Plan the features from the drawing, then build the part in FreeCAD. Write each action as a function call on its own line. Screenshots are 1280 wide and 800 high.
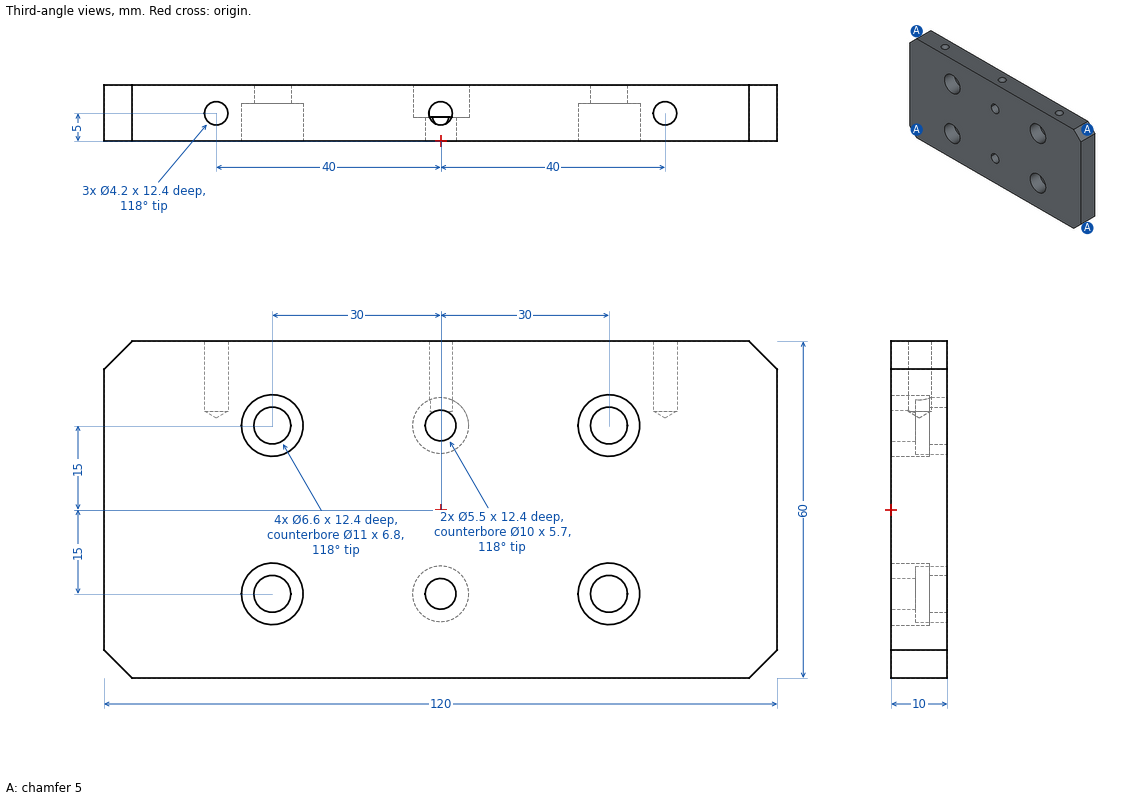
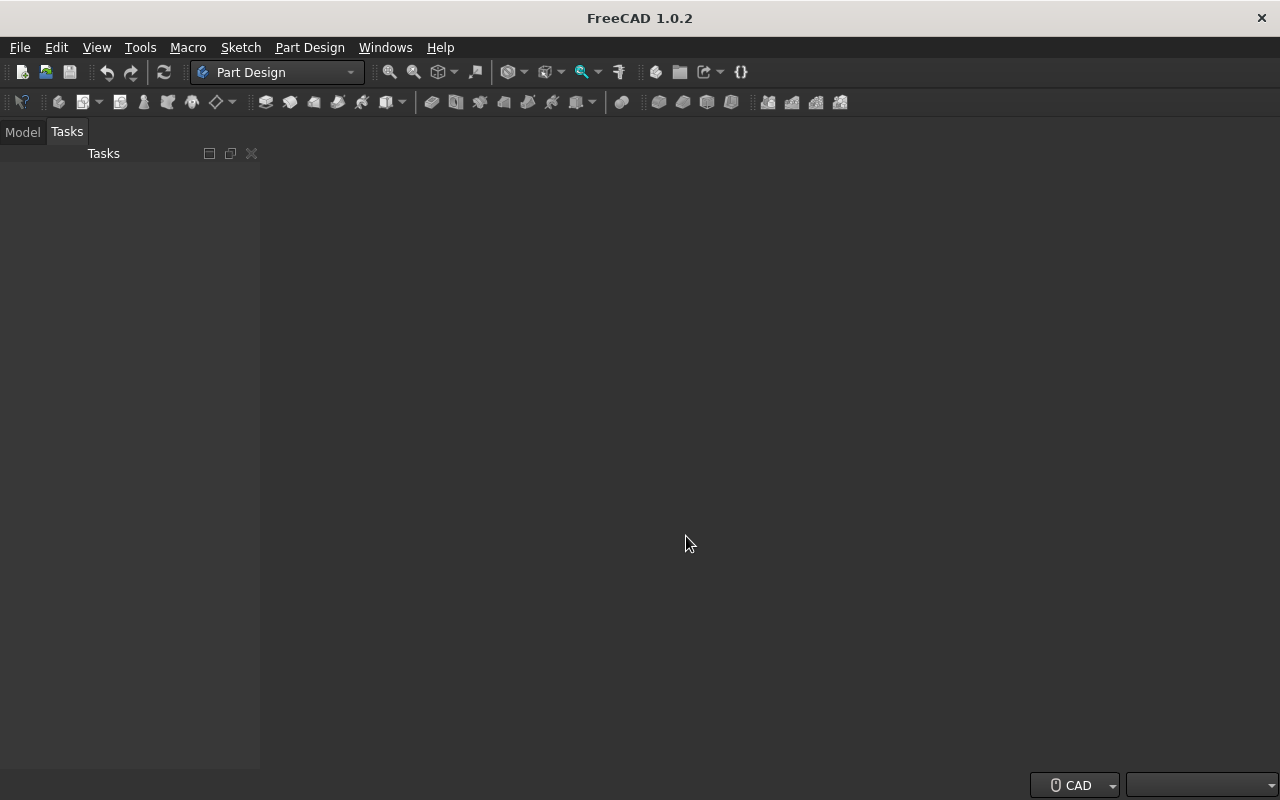
click(22, 72)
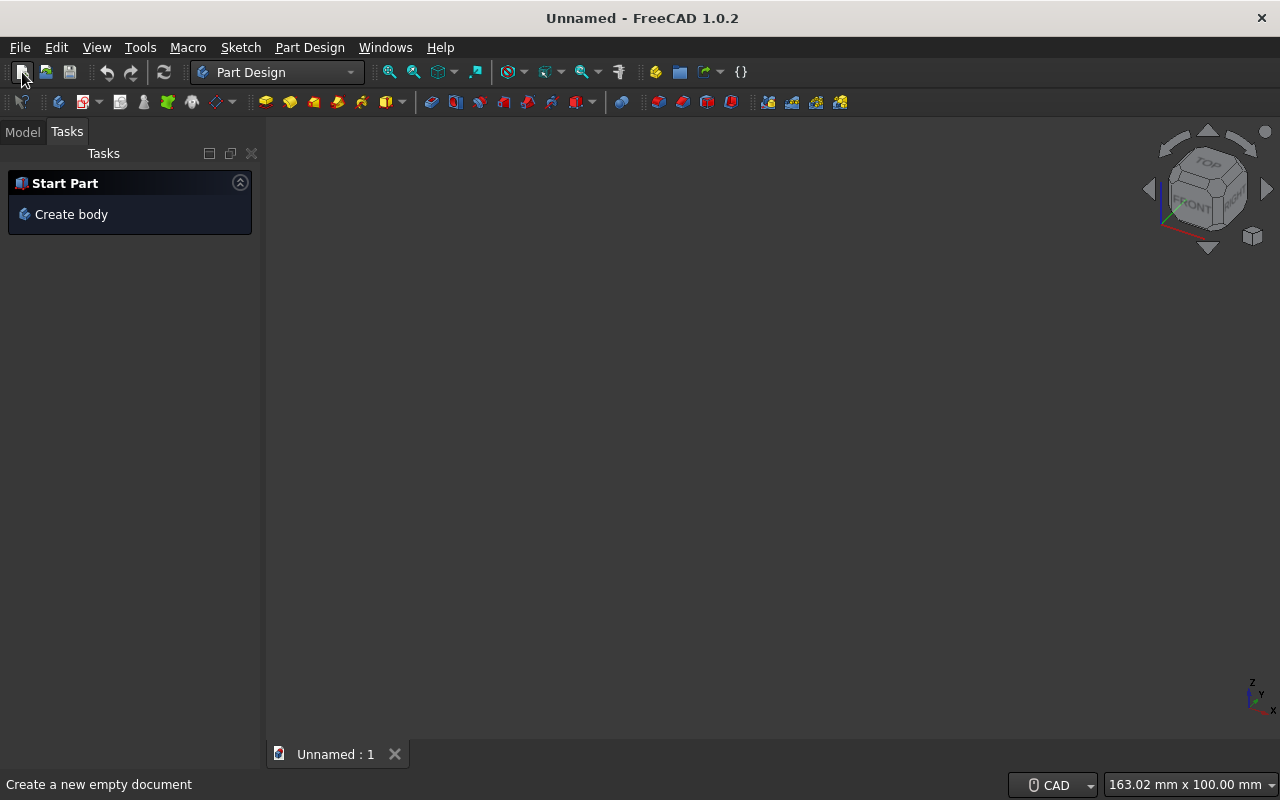
click(84, 102)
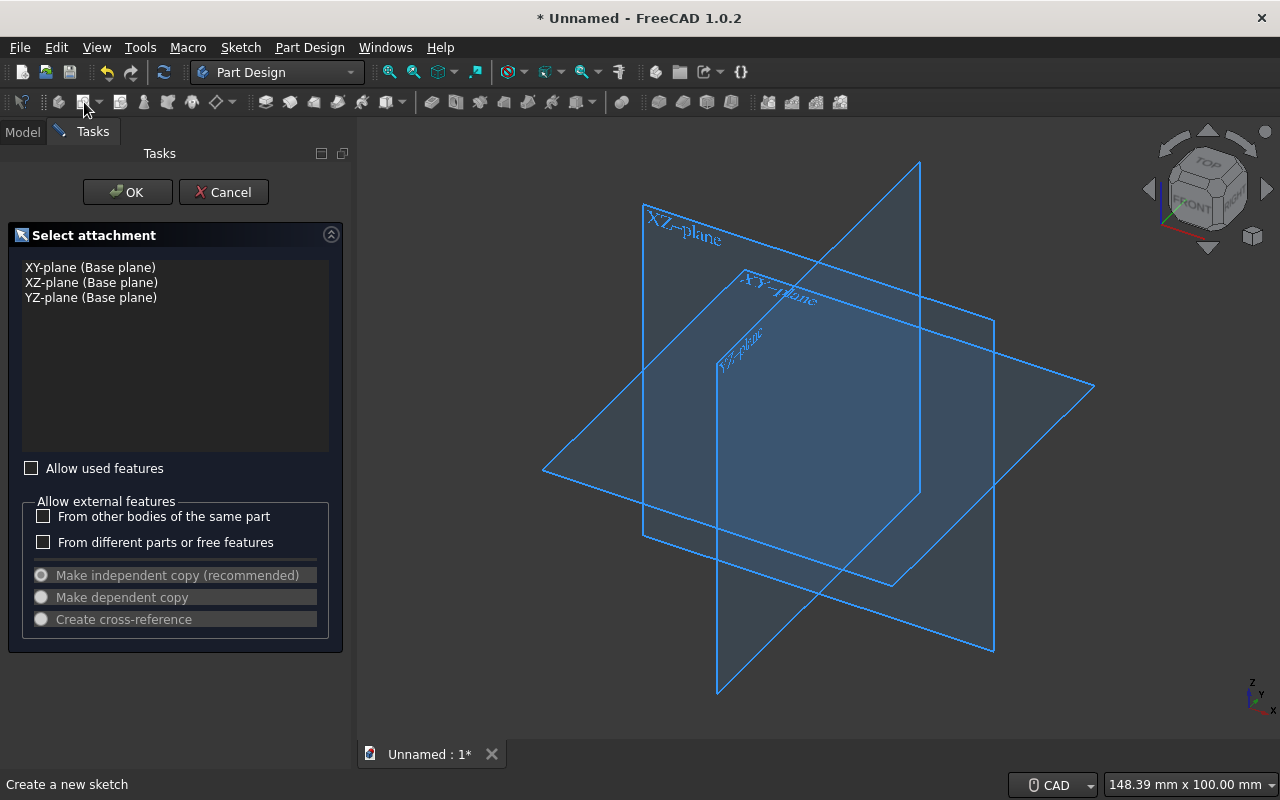
click(82, 282)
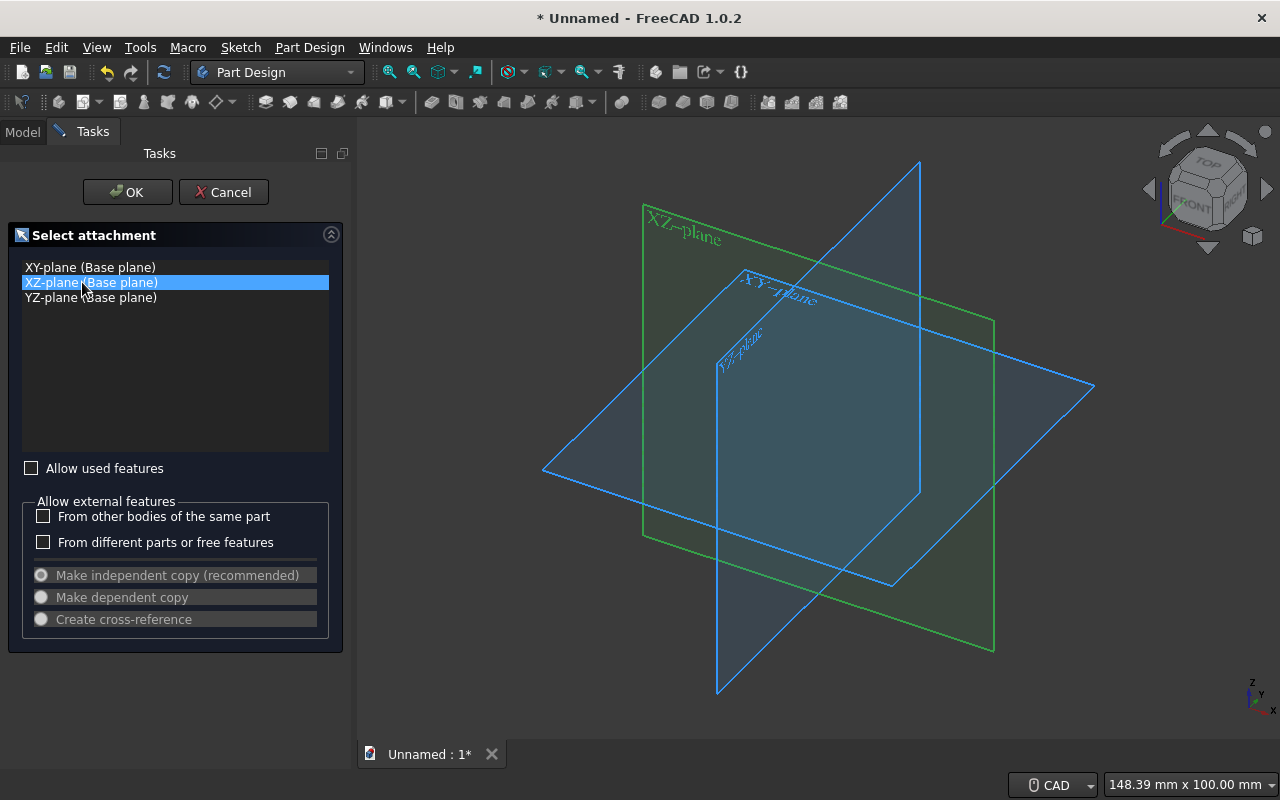
click(128, 192)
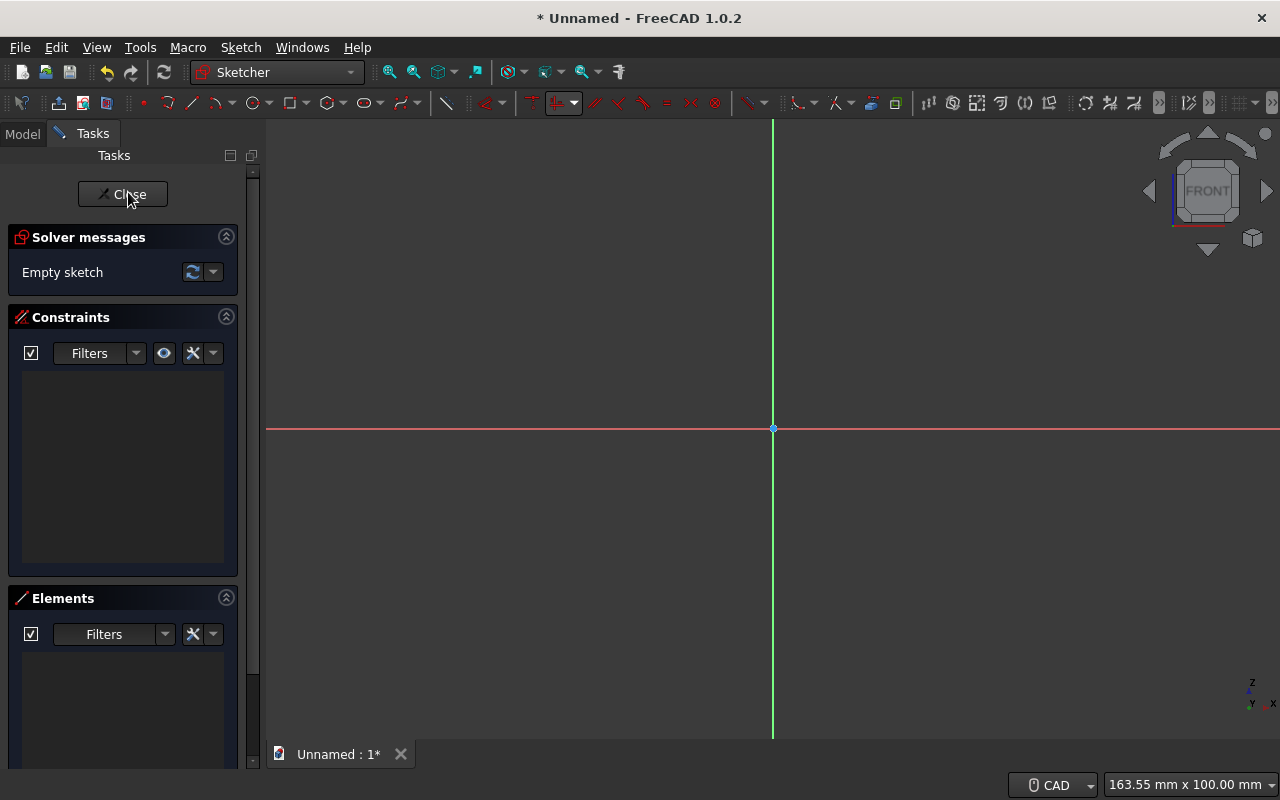
scroll(395, 429, down, 1)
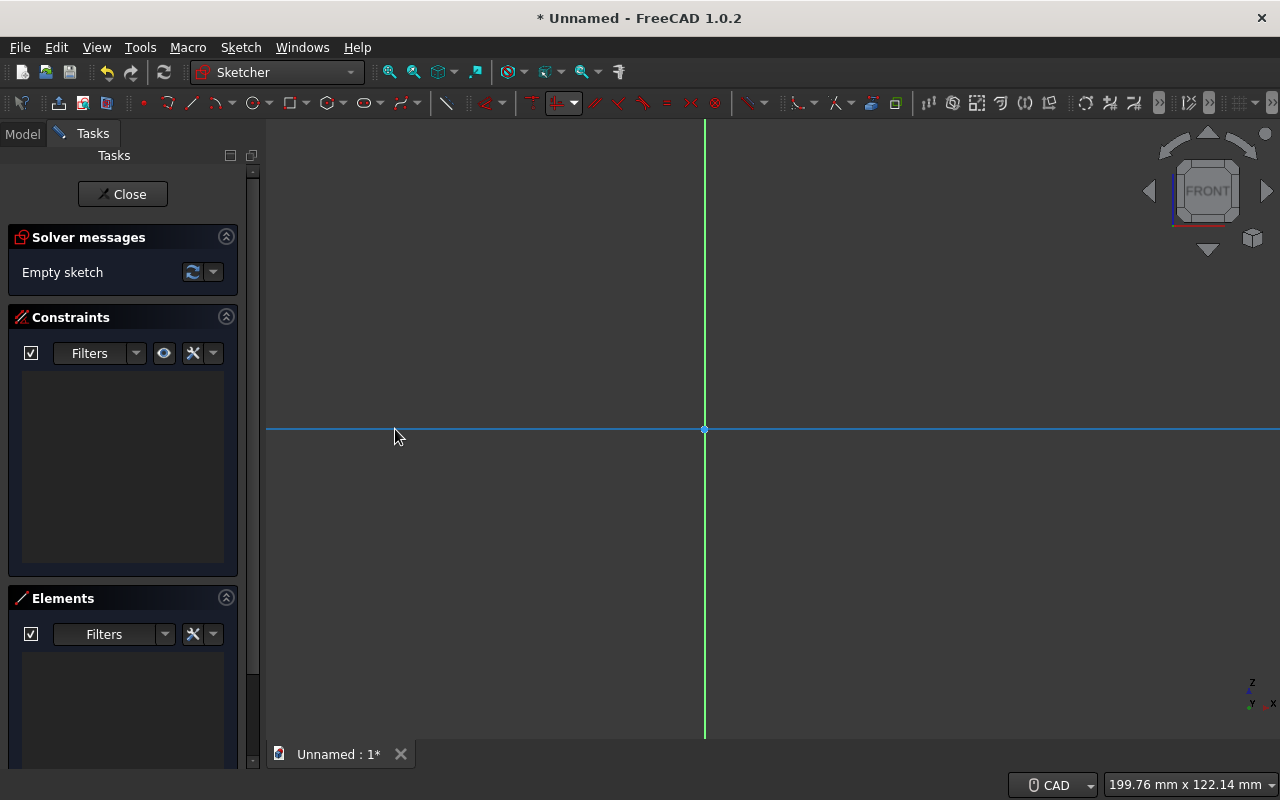
click(308, 104)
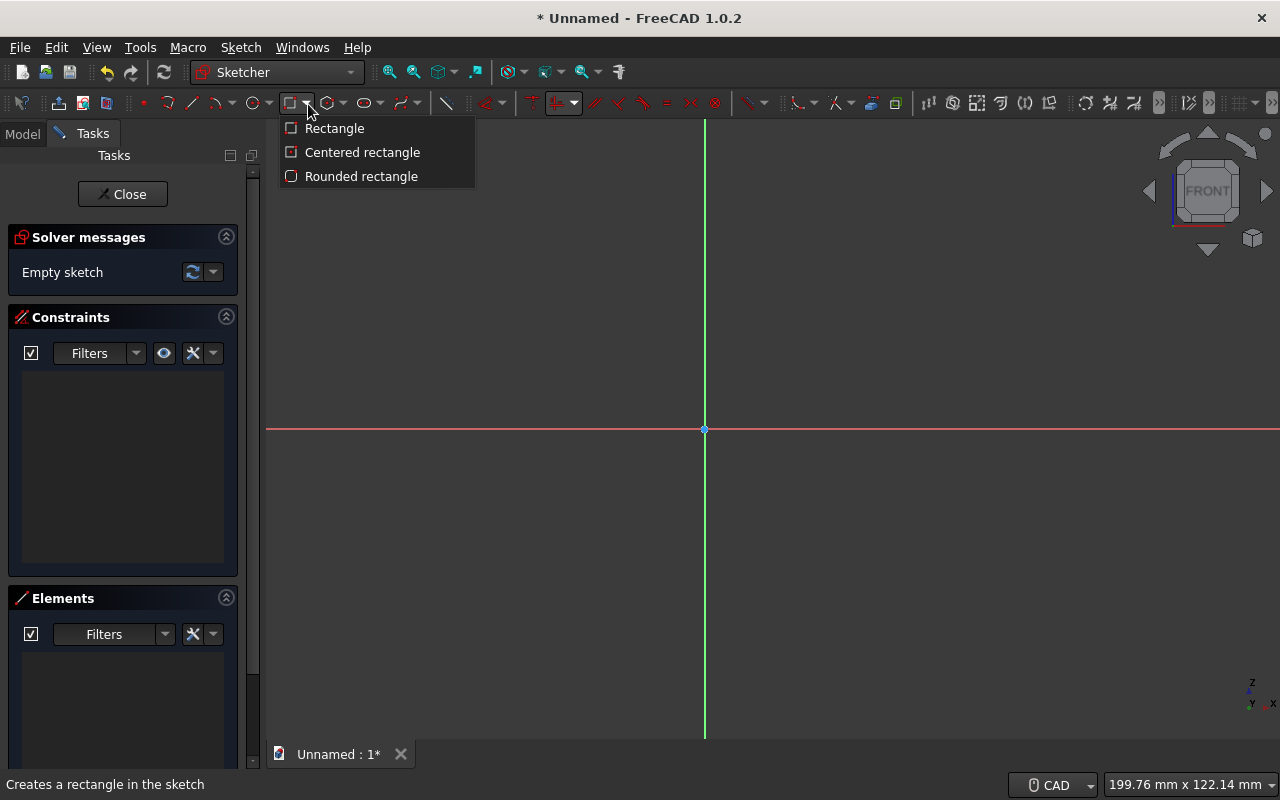
click(378, 152)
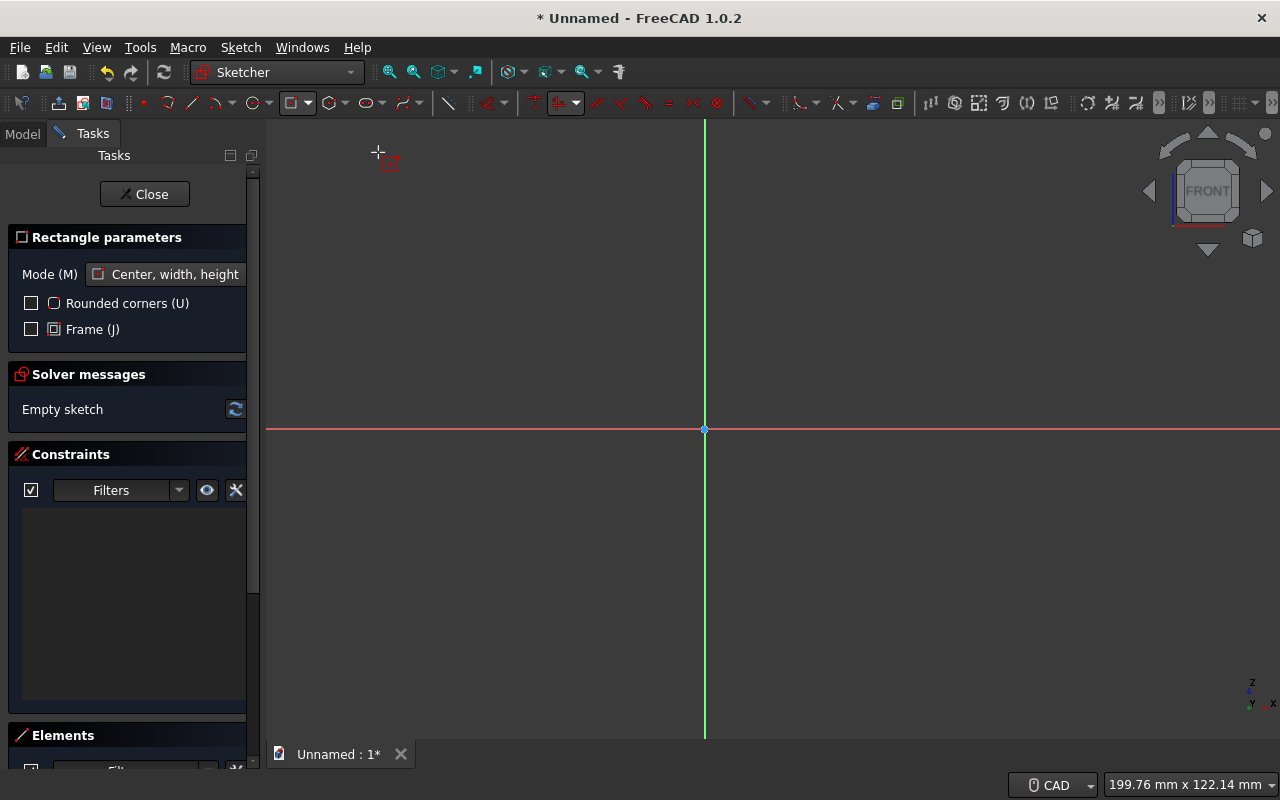
click(705, 429)
move(1009, 277)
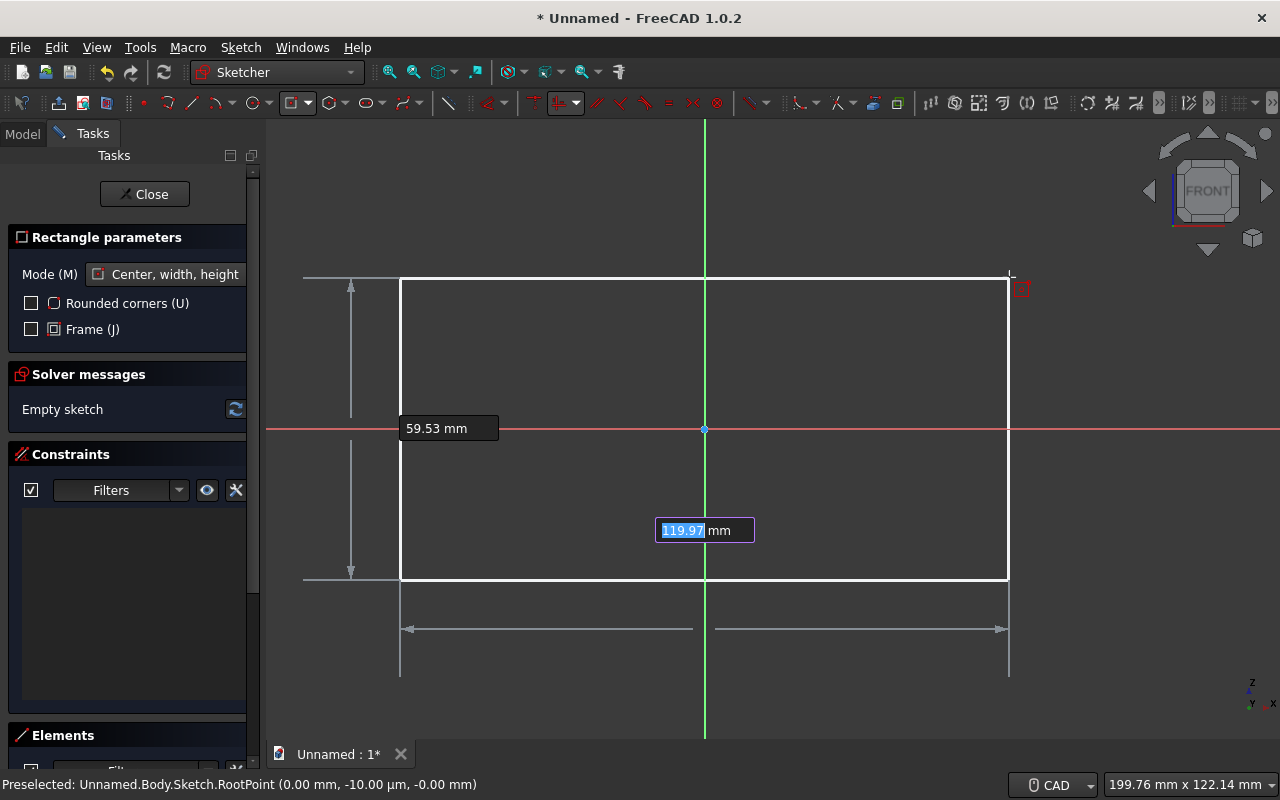
text(120)
key(Tab)
text(60)
key(Return)
key(Escape)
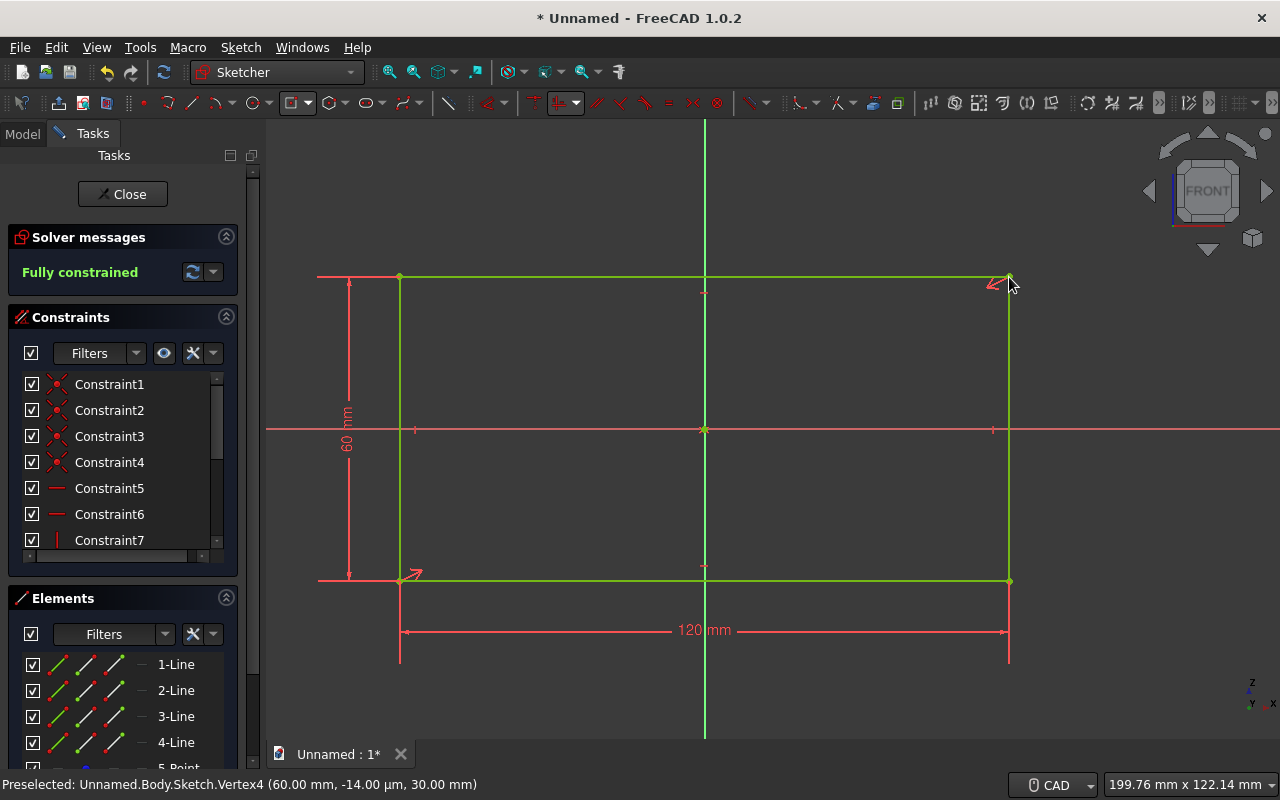
click(123, 194)